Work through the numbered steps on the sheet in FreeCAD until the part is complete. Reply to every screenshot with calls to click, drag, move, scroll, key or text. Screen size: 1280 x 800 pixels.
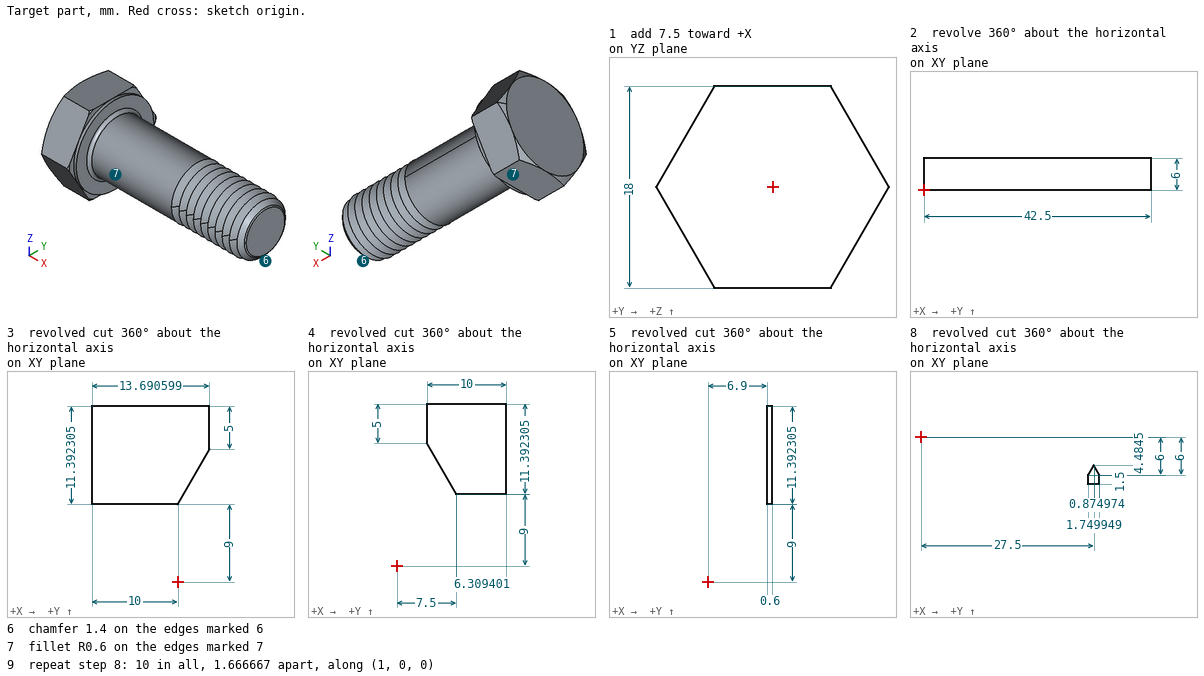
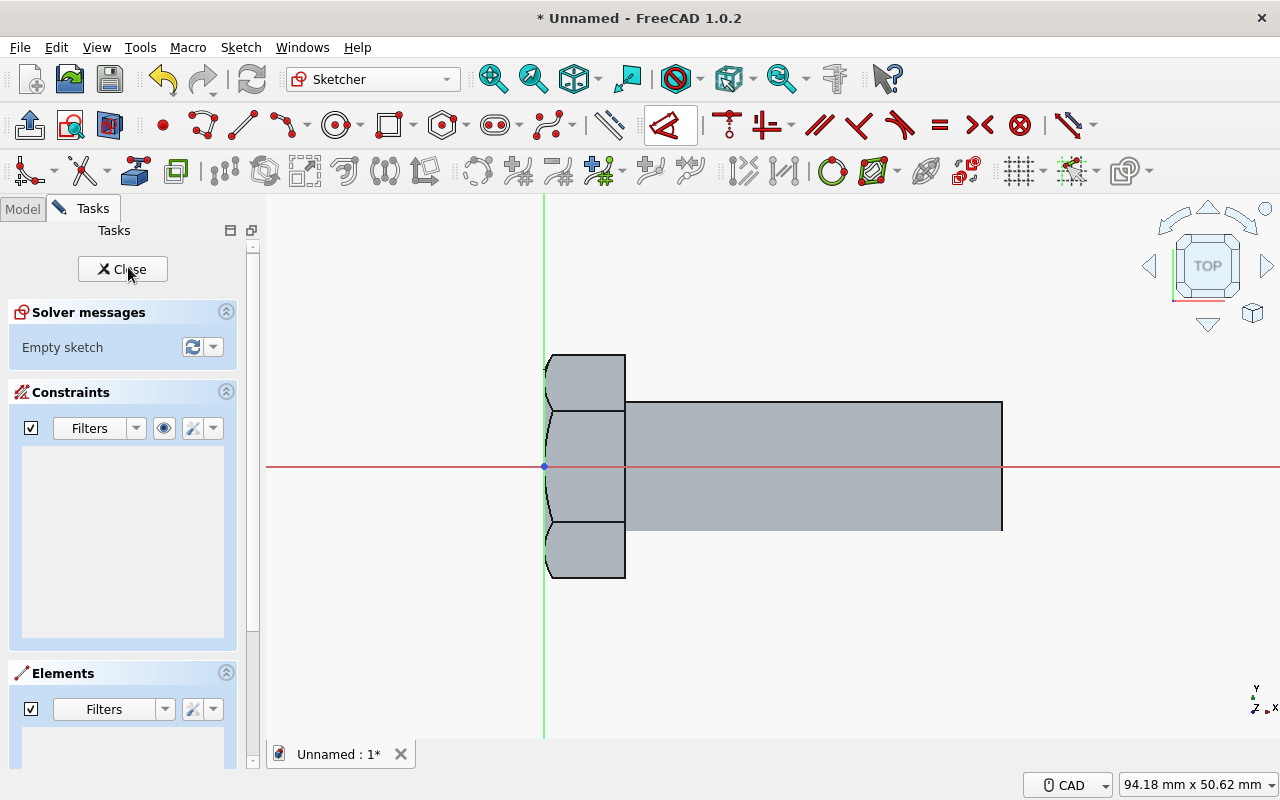
scroll(444, 222, up, 2)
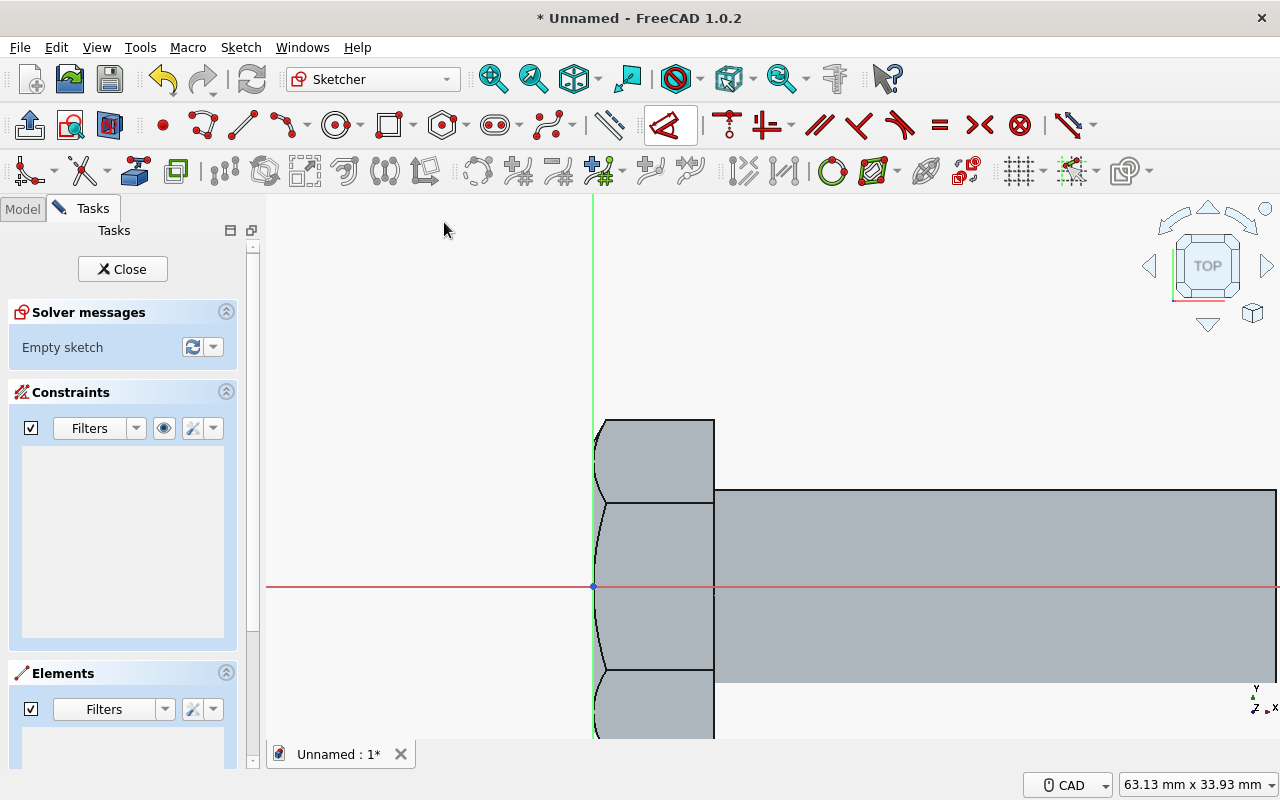
key(g)
key(m)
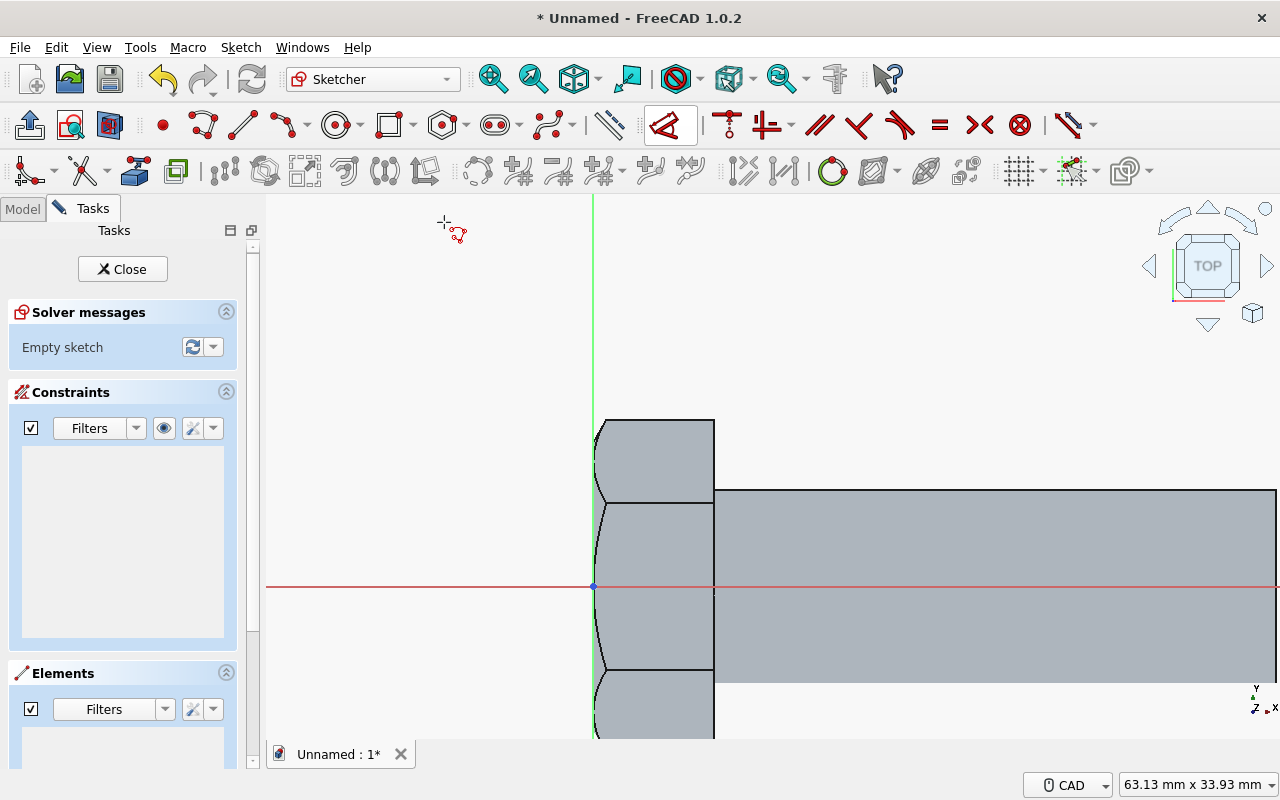
click(714, 442)
click(815, 442)
click(815, 259)
click(655, 259)
click(655, 339)
click(714, 443)
key(Escape)
key(Escape)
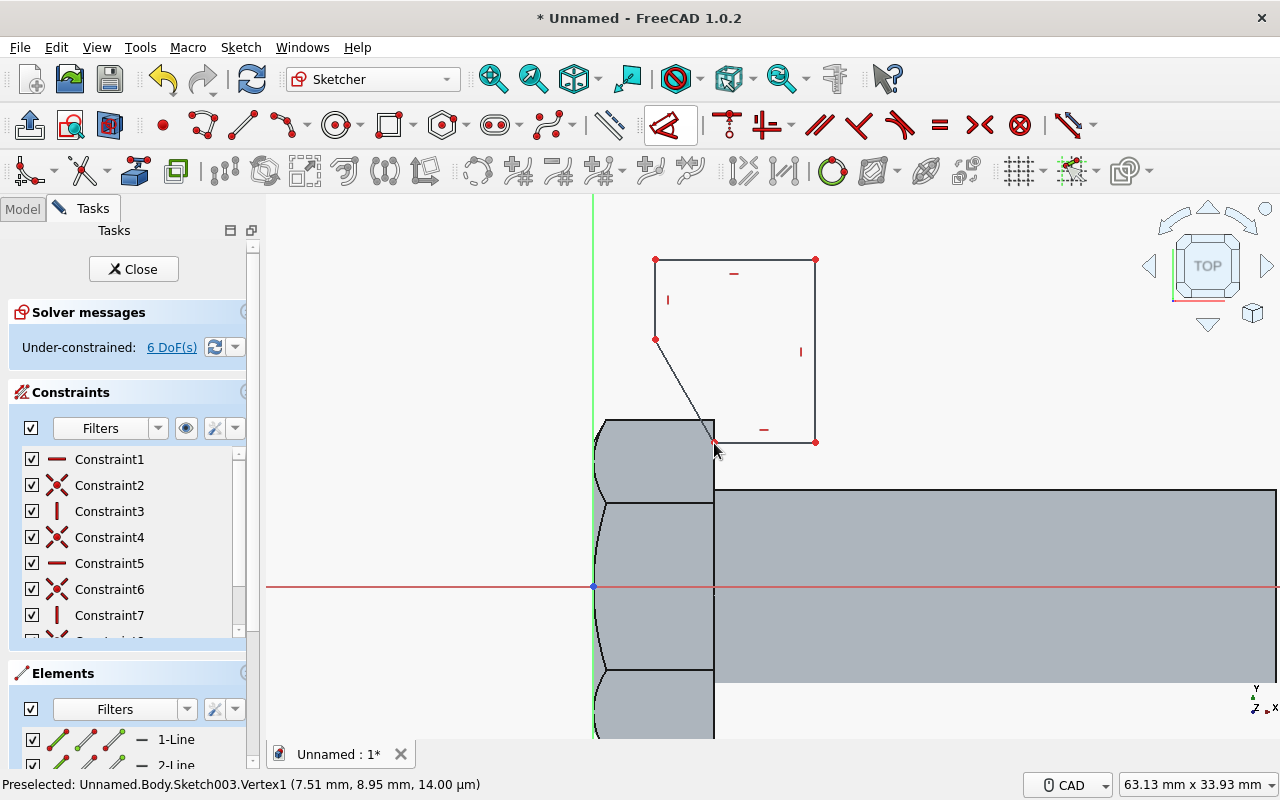
click(655, 284)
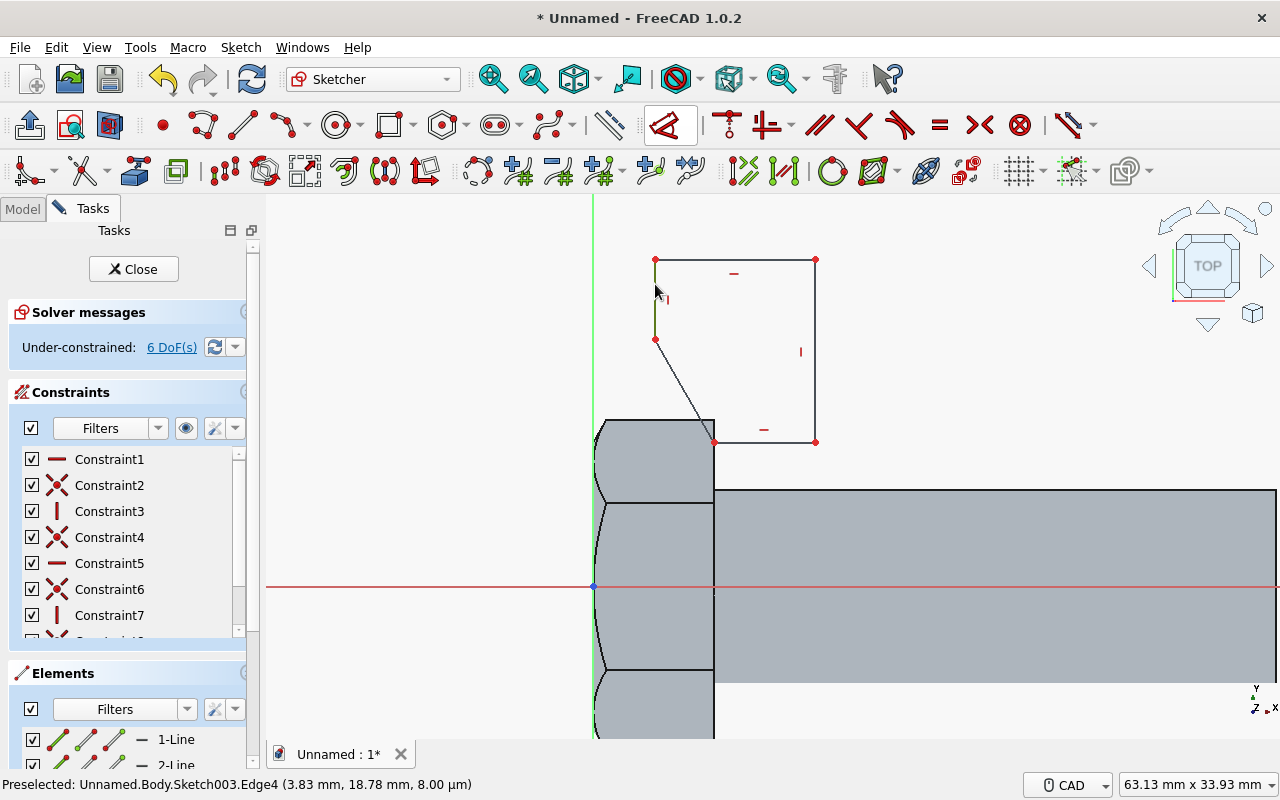
click(692, 126)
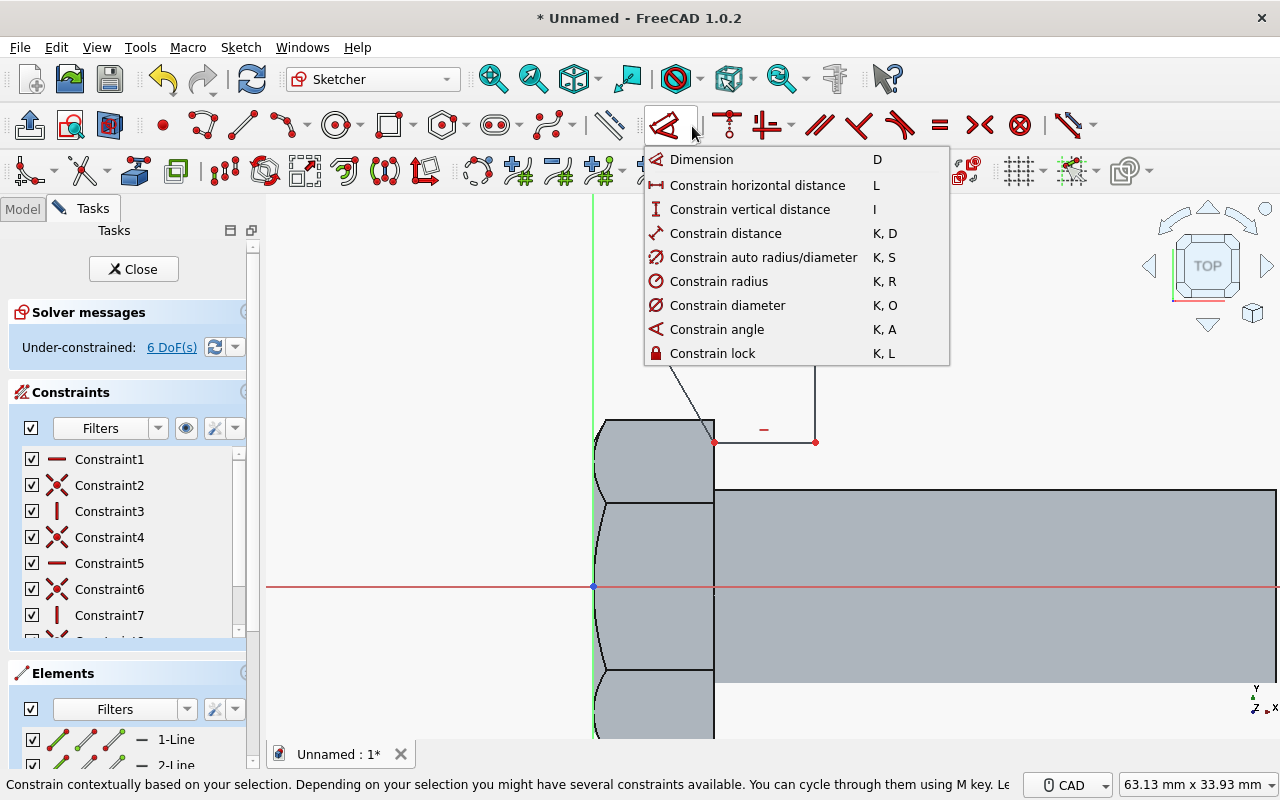
click(797, 209)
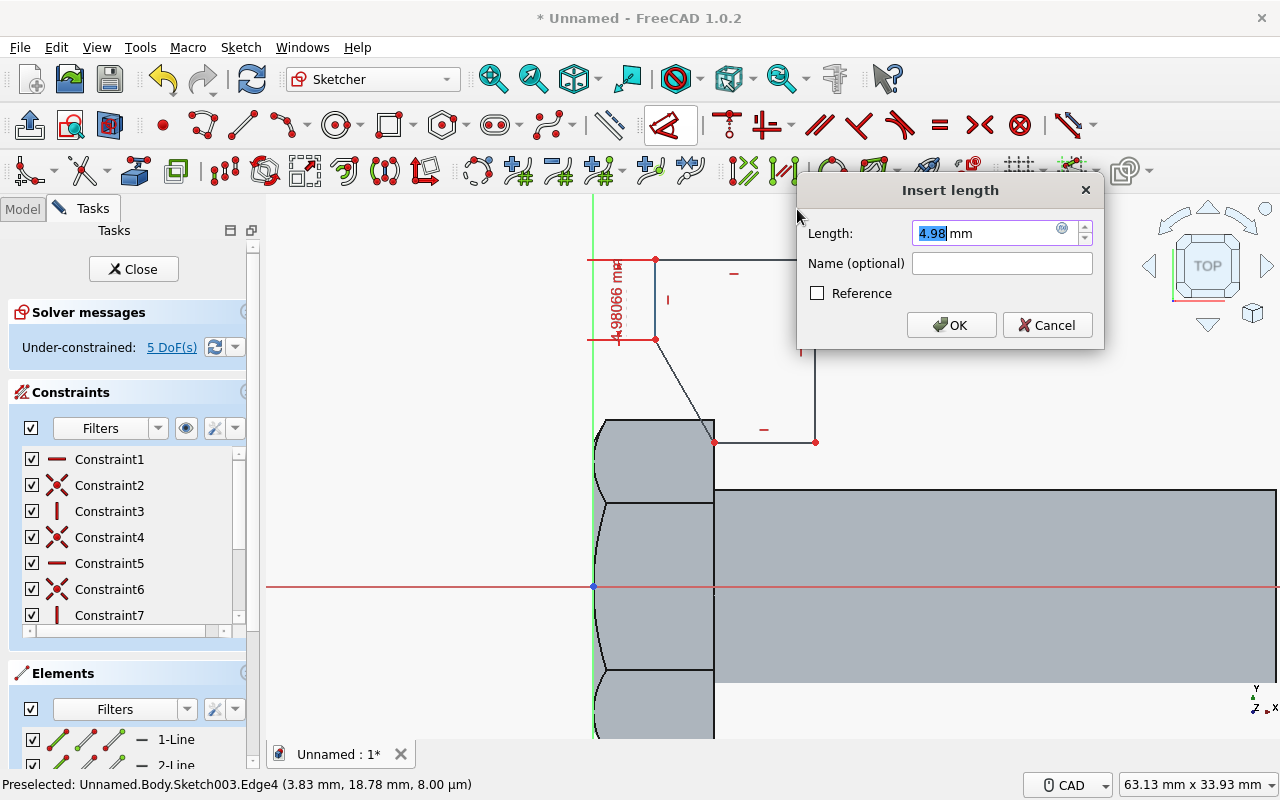
text(5)
key(Return)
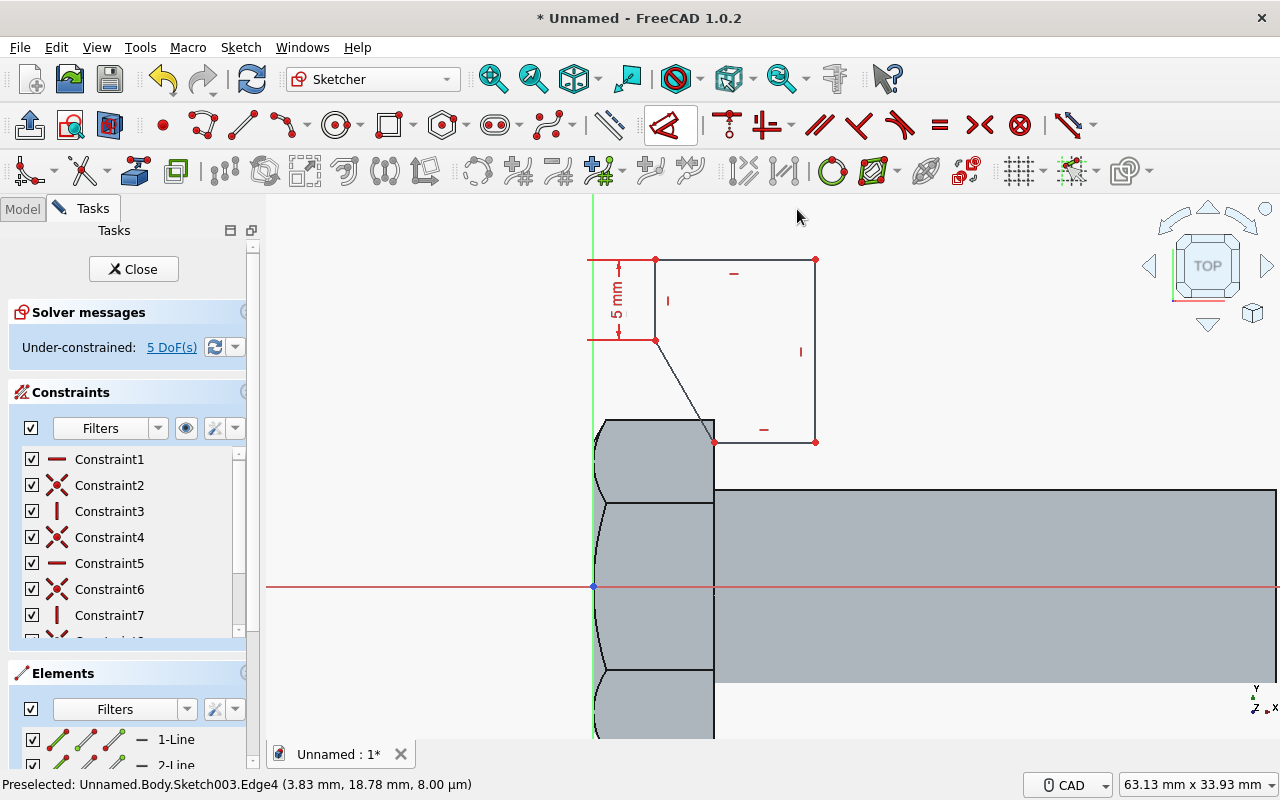
click(767, 260)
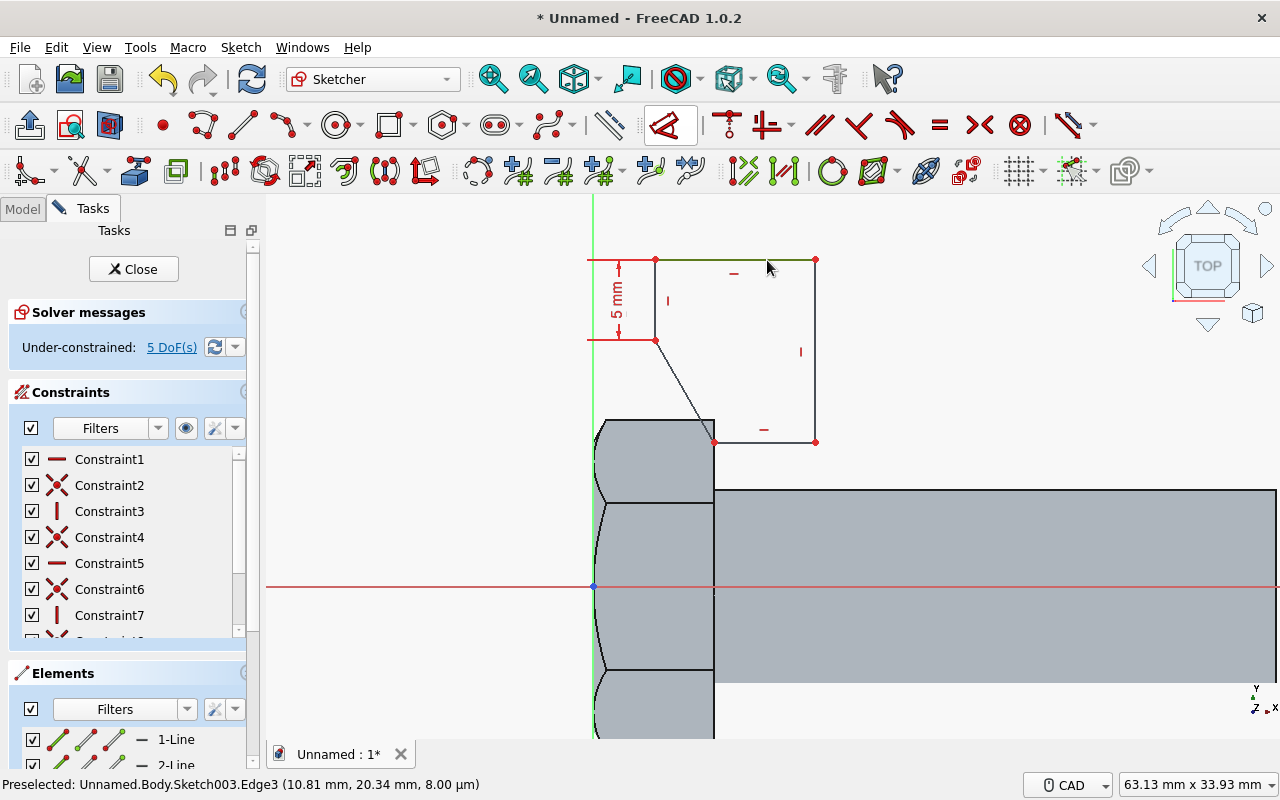
click(692, 126)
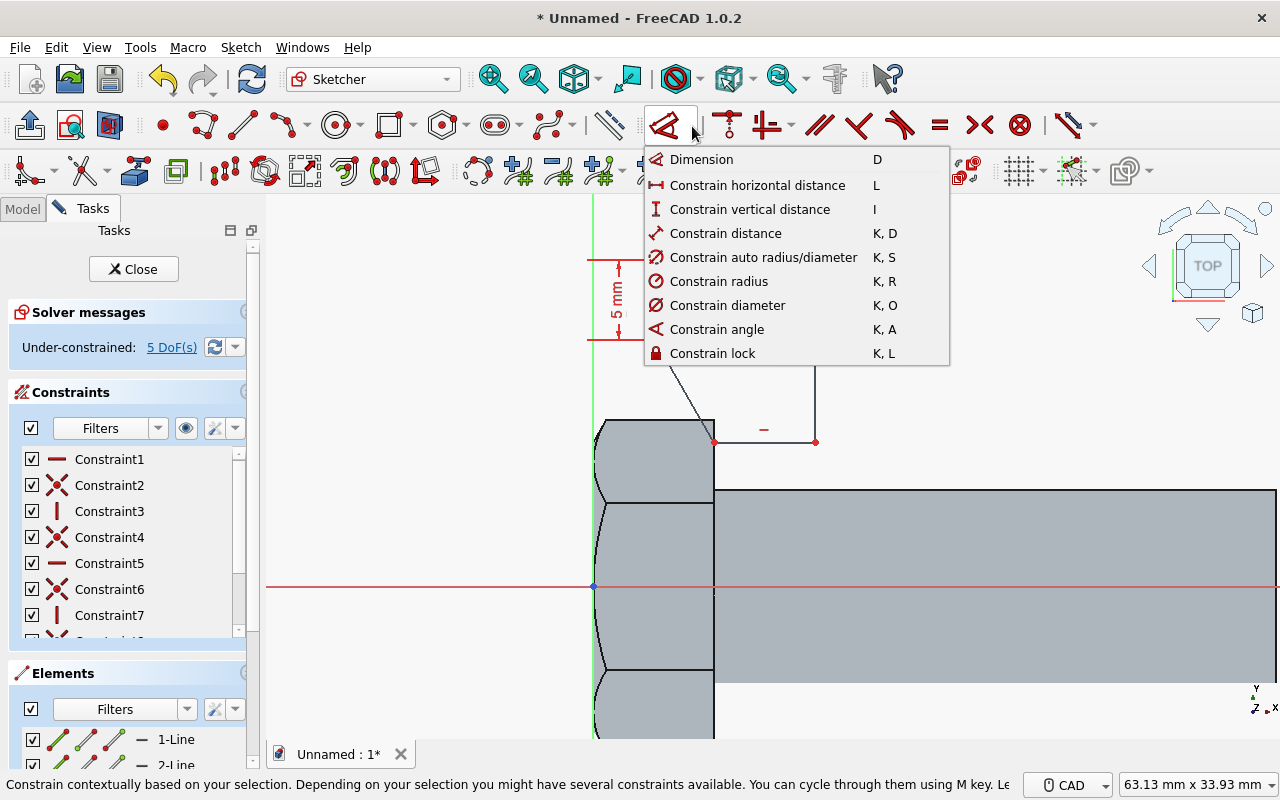
click(797, 185)